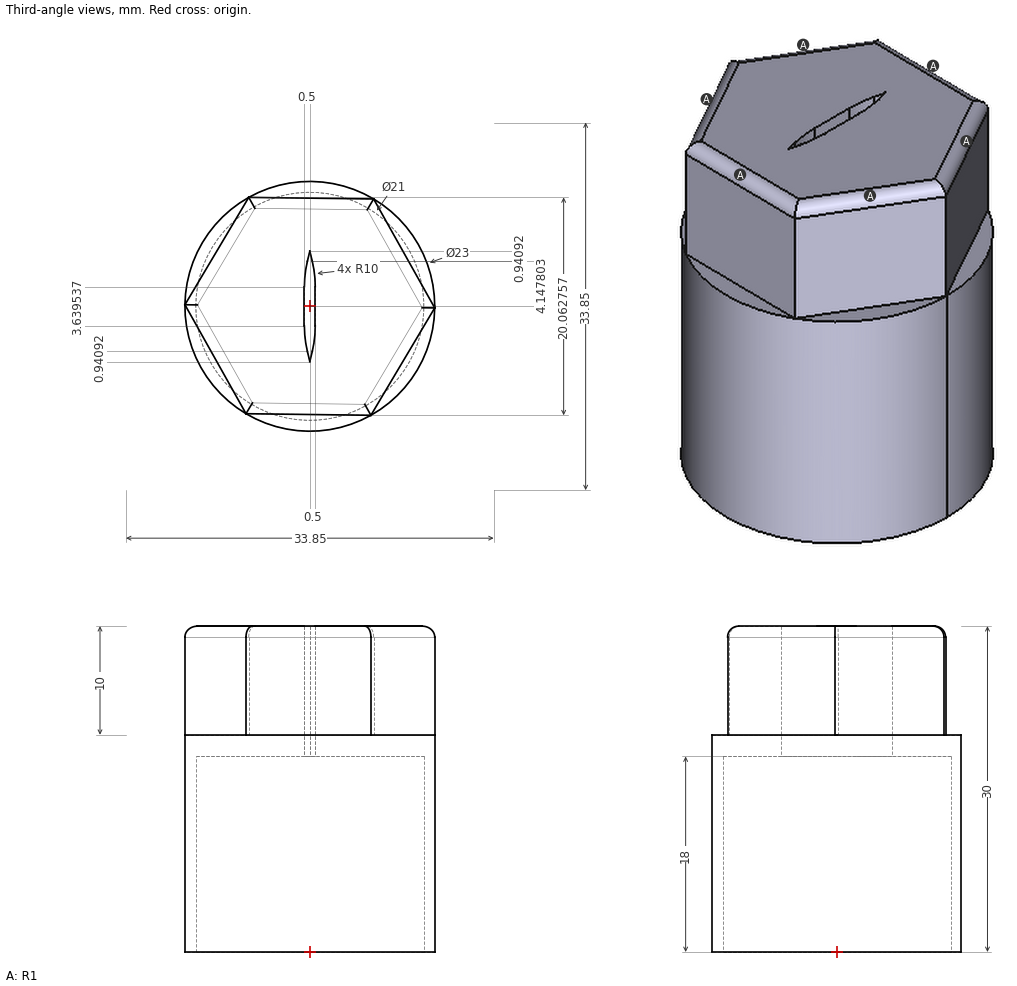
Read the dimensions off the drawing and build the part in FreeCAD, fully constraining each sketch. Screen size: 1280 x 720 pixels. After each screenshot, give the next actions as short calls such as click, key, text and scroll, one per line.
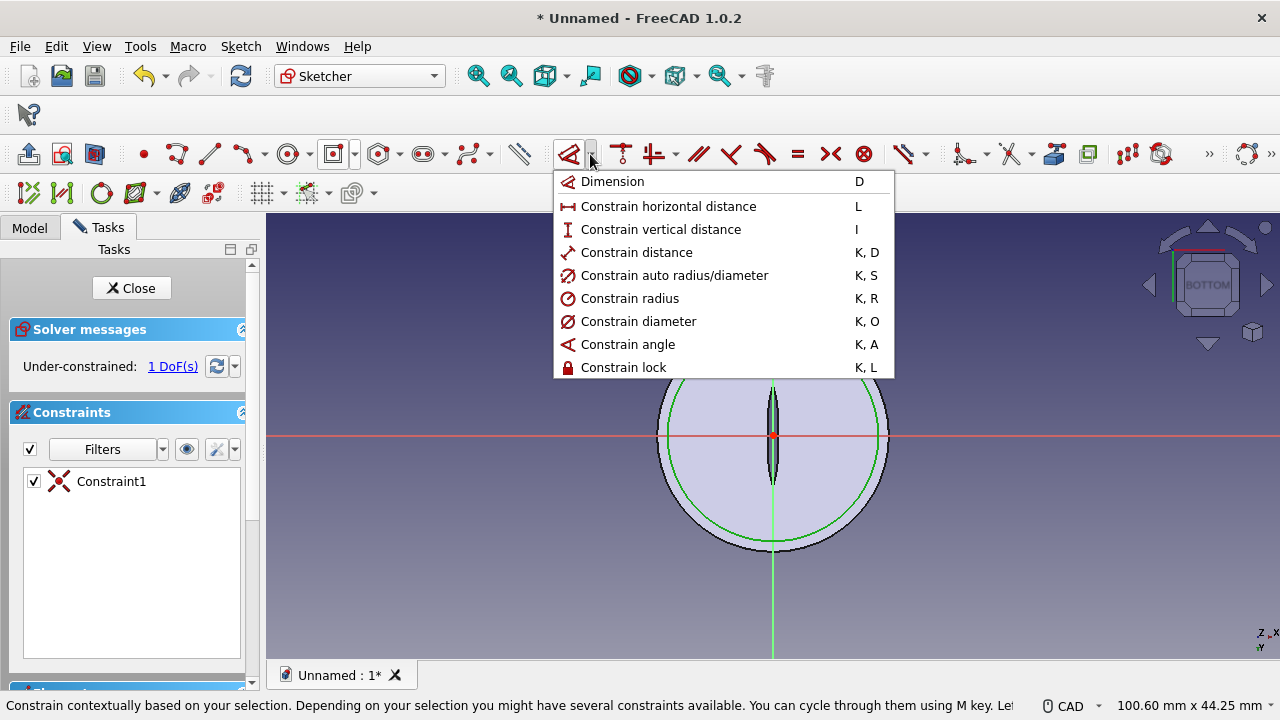
click(724, 322)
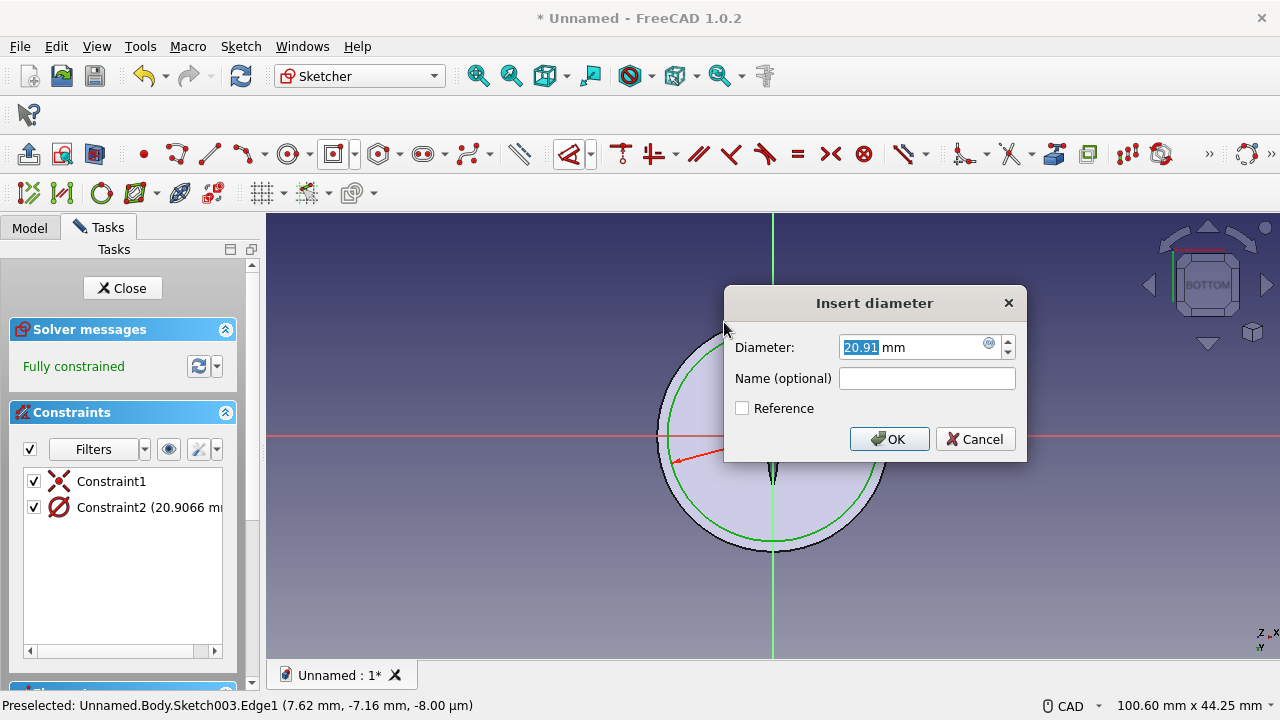
text(21)
key(Return)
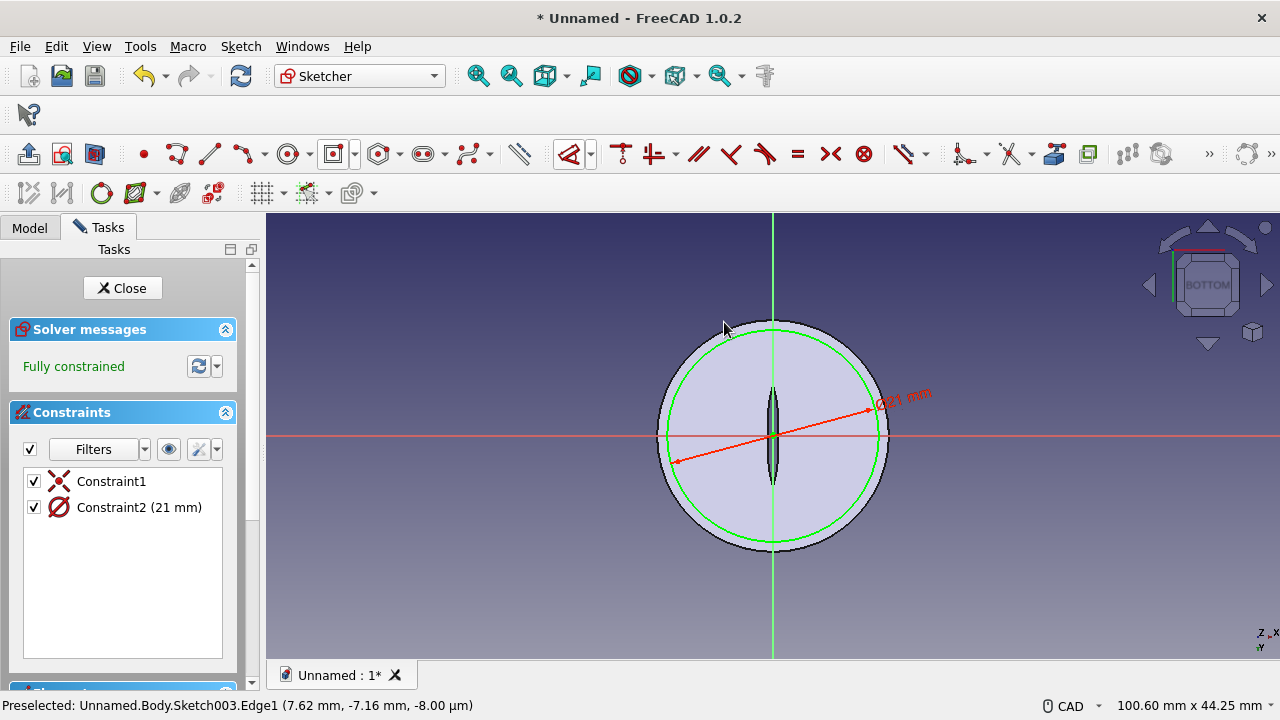
click(123, 288)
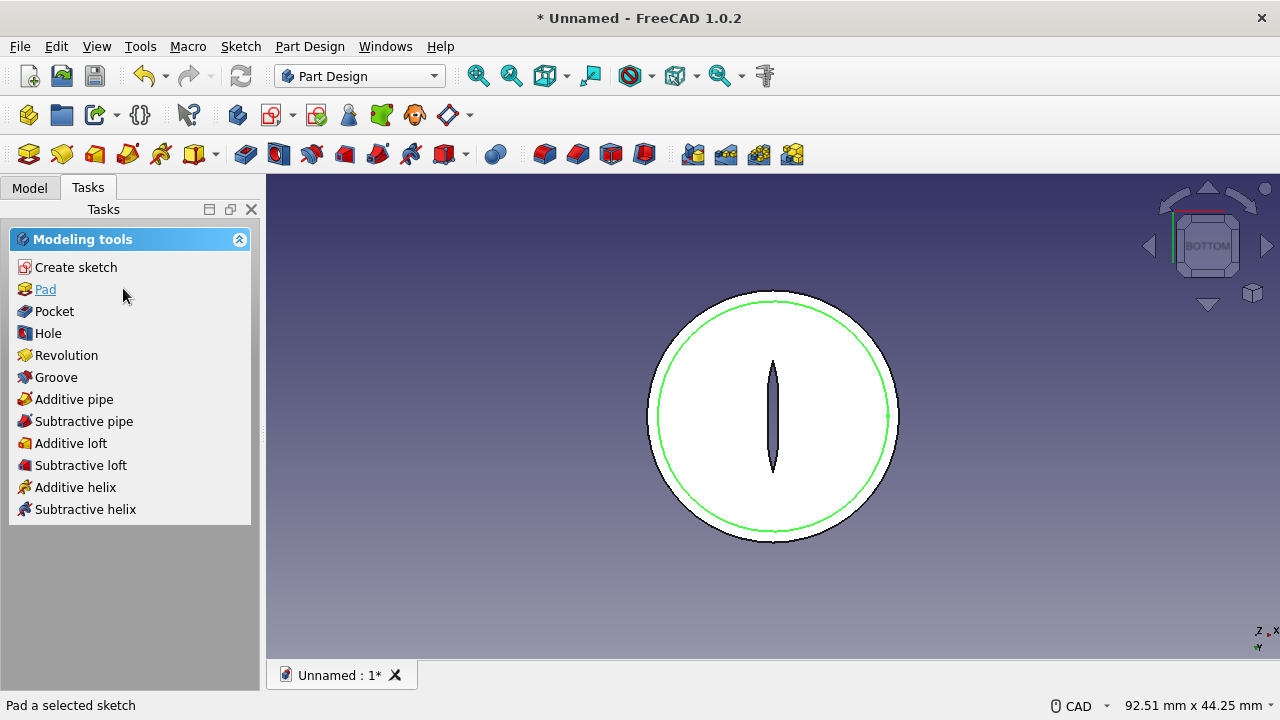
click(246, 154)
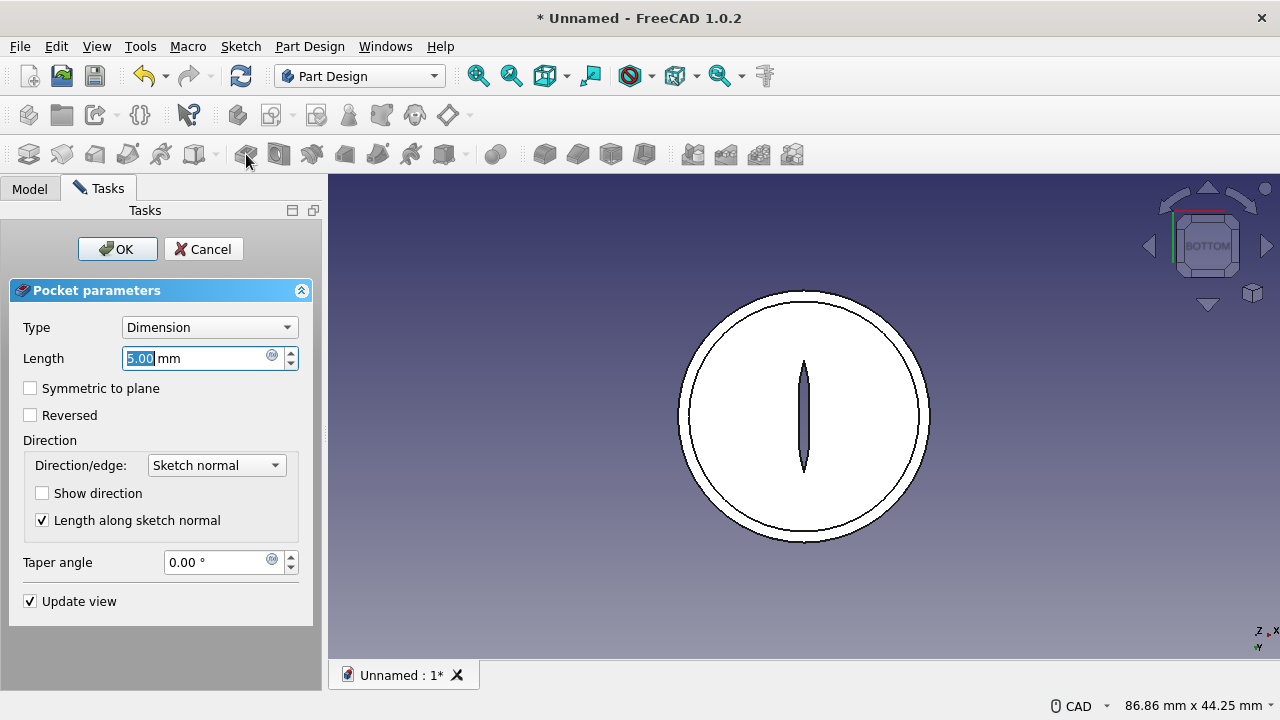
text(18)
key(Tab)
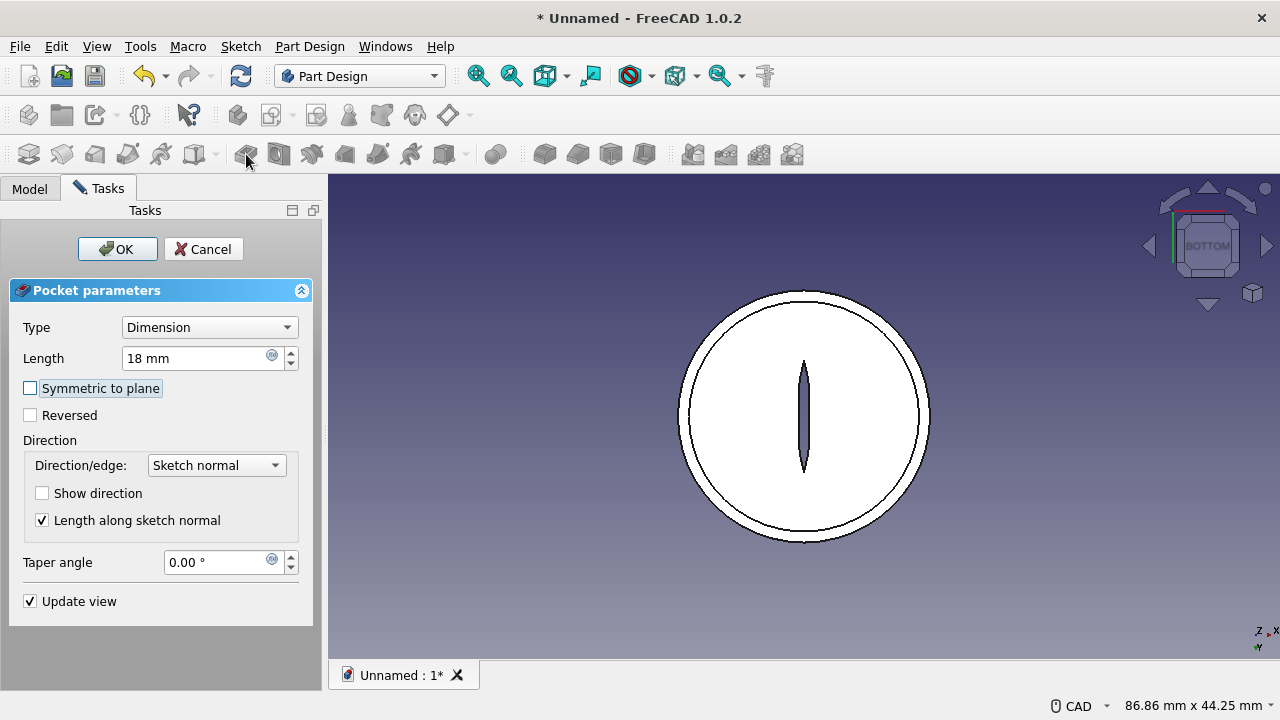
click(118, 249)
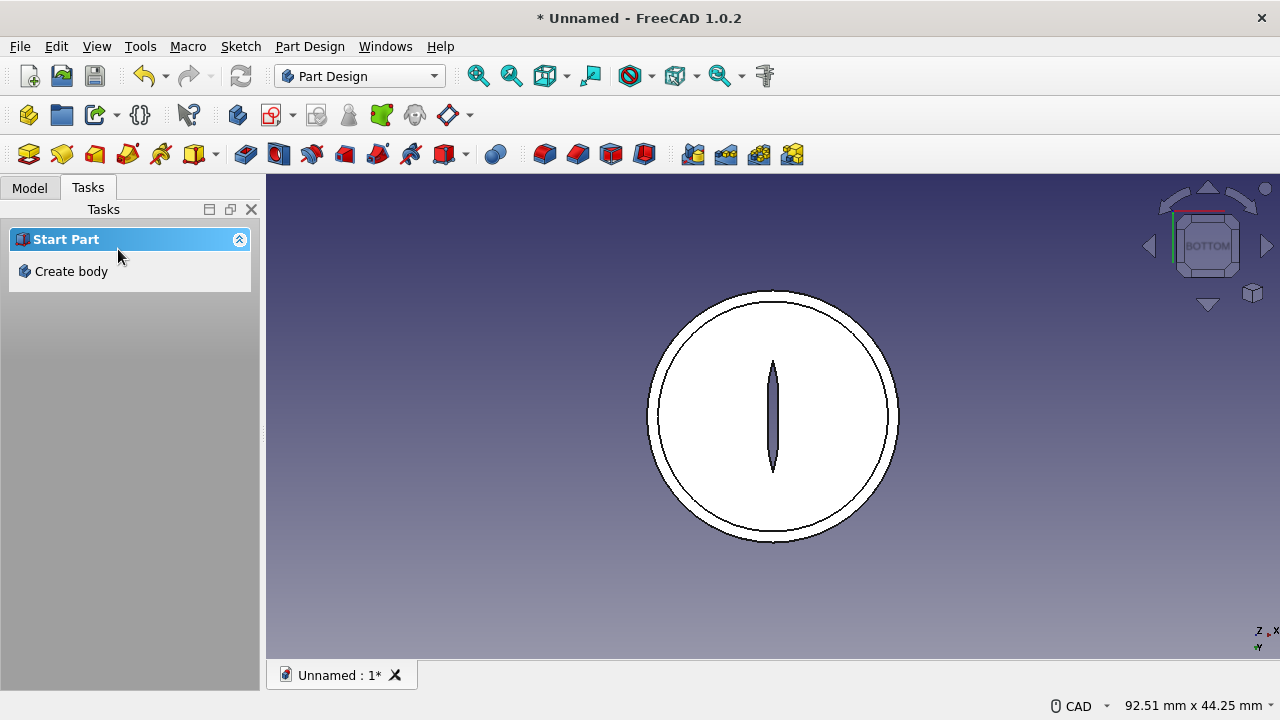
key(0)